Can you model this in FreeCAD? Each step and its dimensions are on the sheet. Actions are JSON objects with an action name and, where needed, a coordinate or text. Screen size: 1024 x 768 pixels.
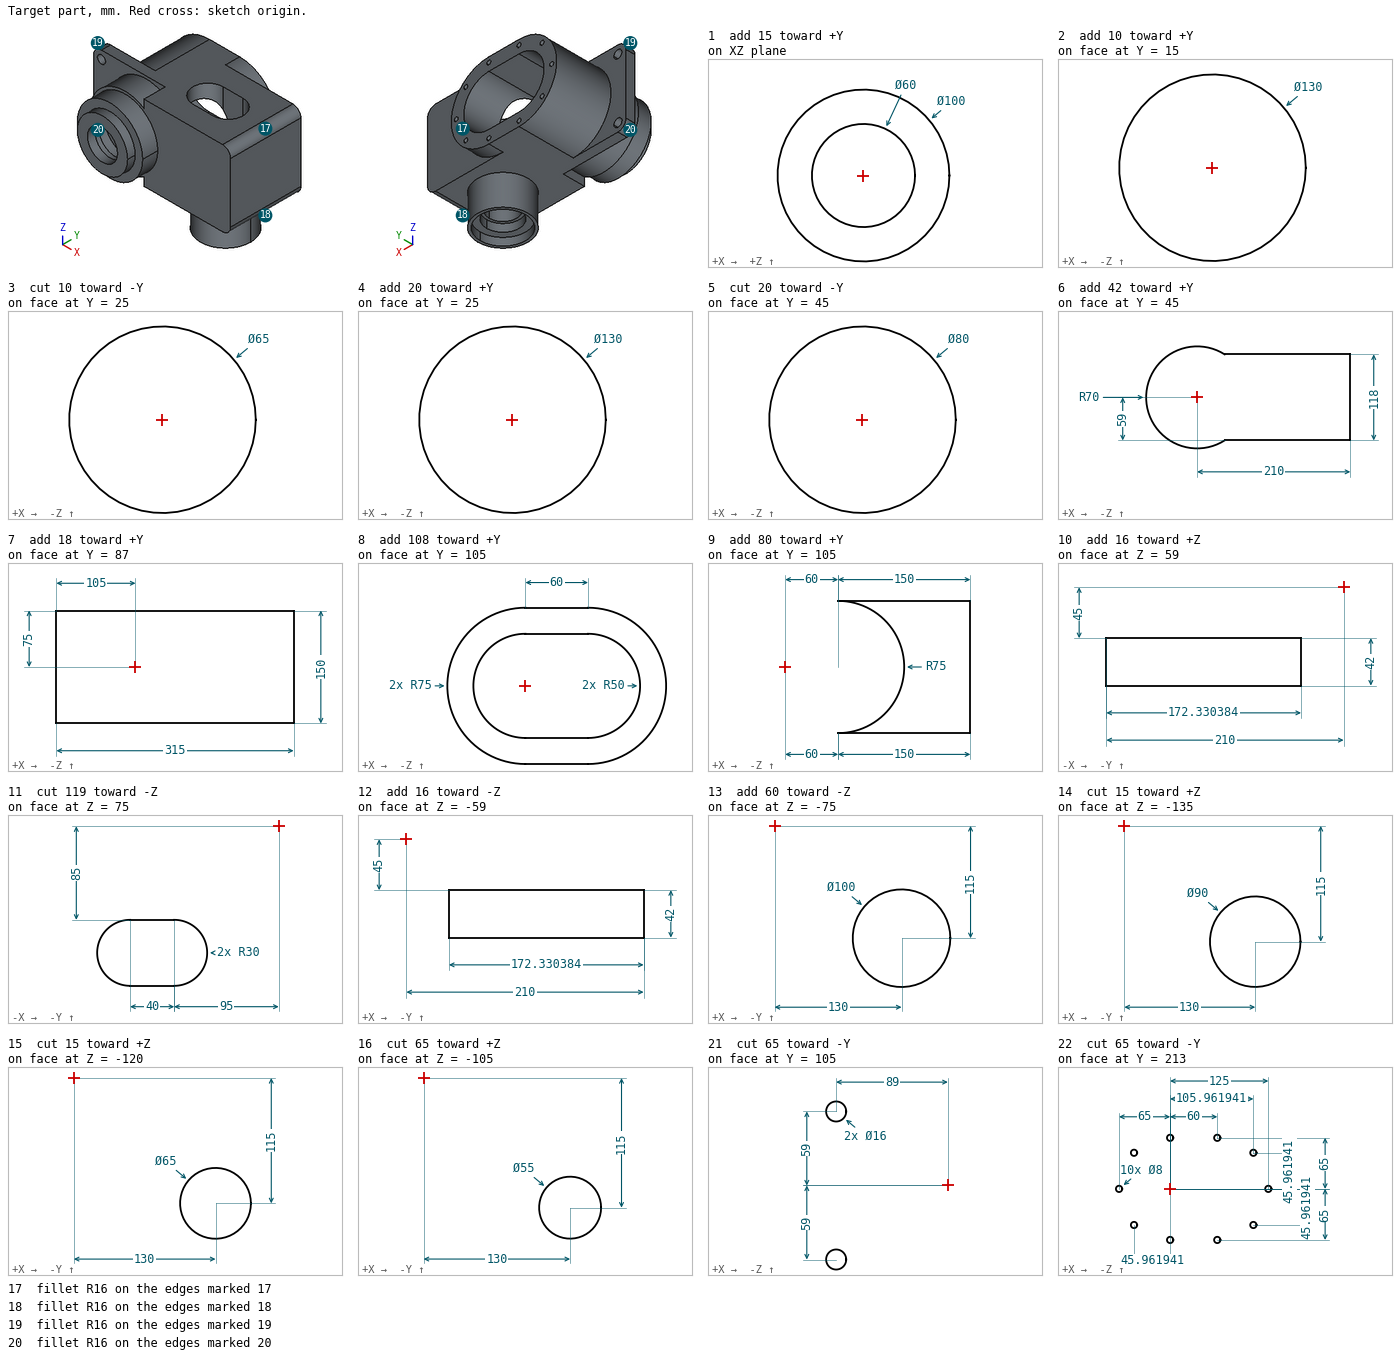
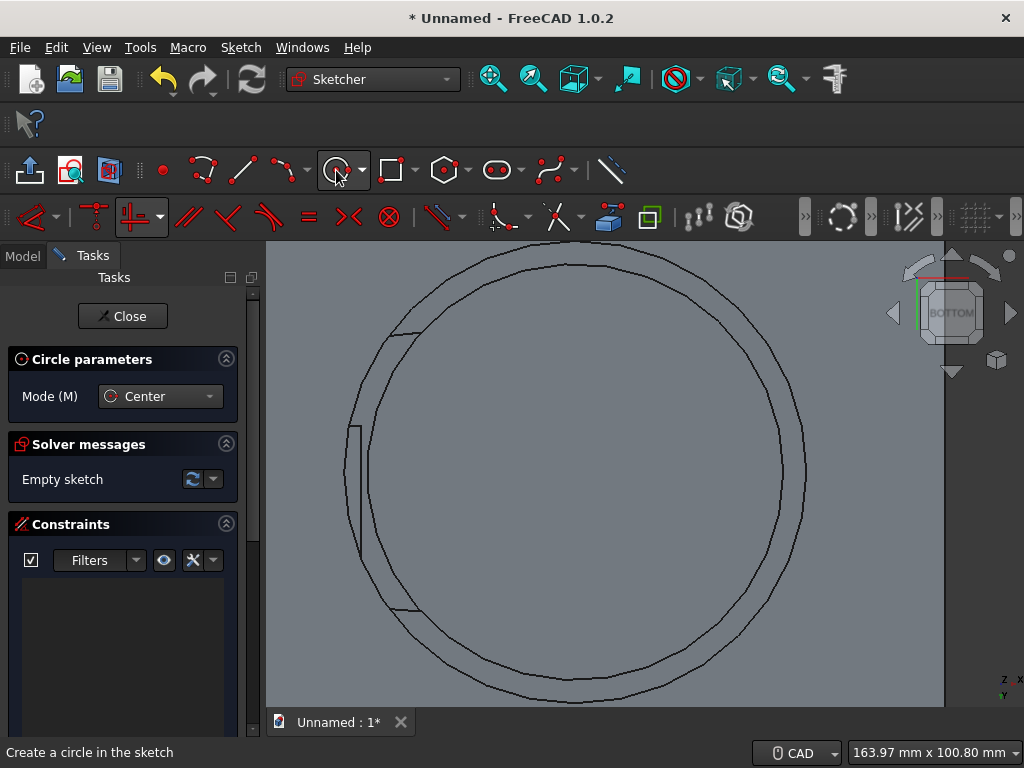
{"action": "left_click", "coordinate": [575, 472]}
{"action": "mouse_move", "coordinate": [682, 366]}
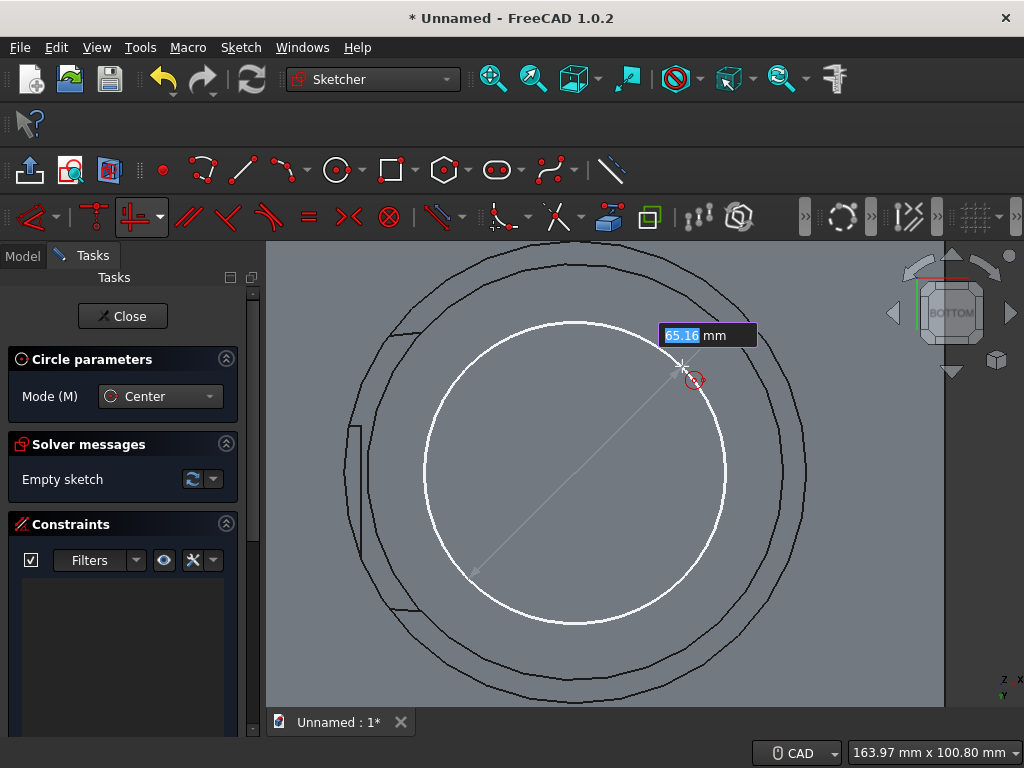
{"action": "type", "text": "65"}
{"action": "key", "text": "Return"}
{"action": "key", "text": "Escape"}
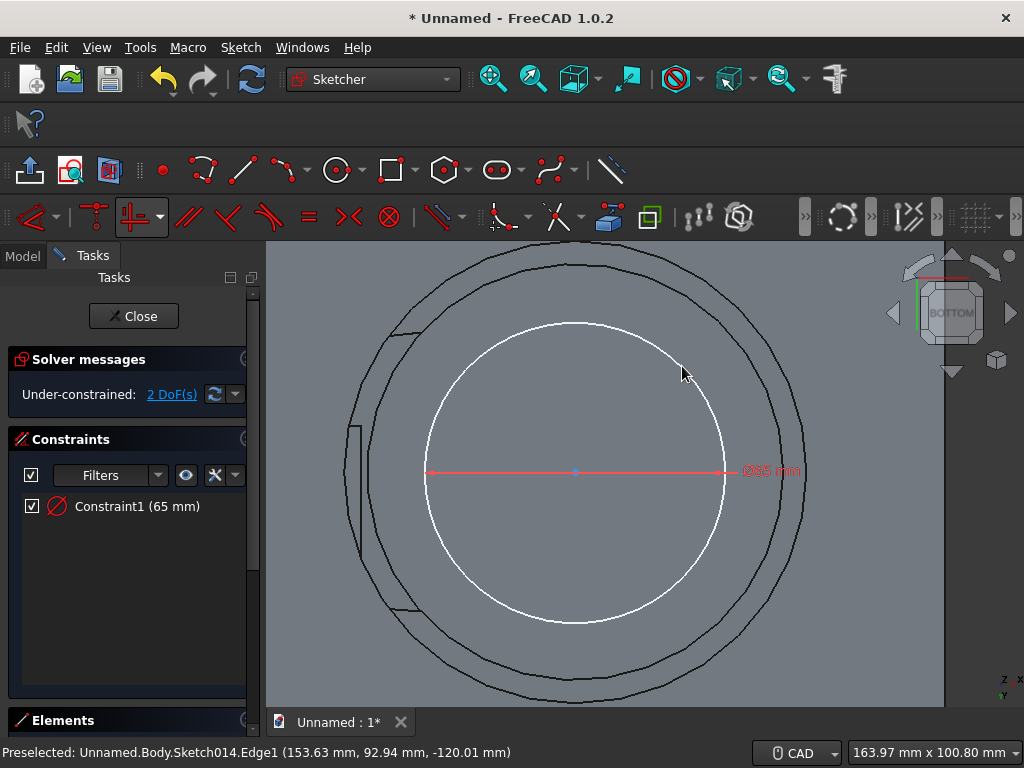
{"action": "left_click", "coordinate": [32, 218]}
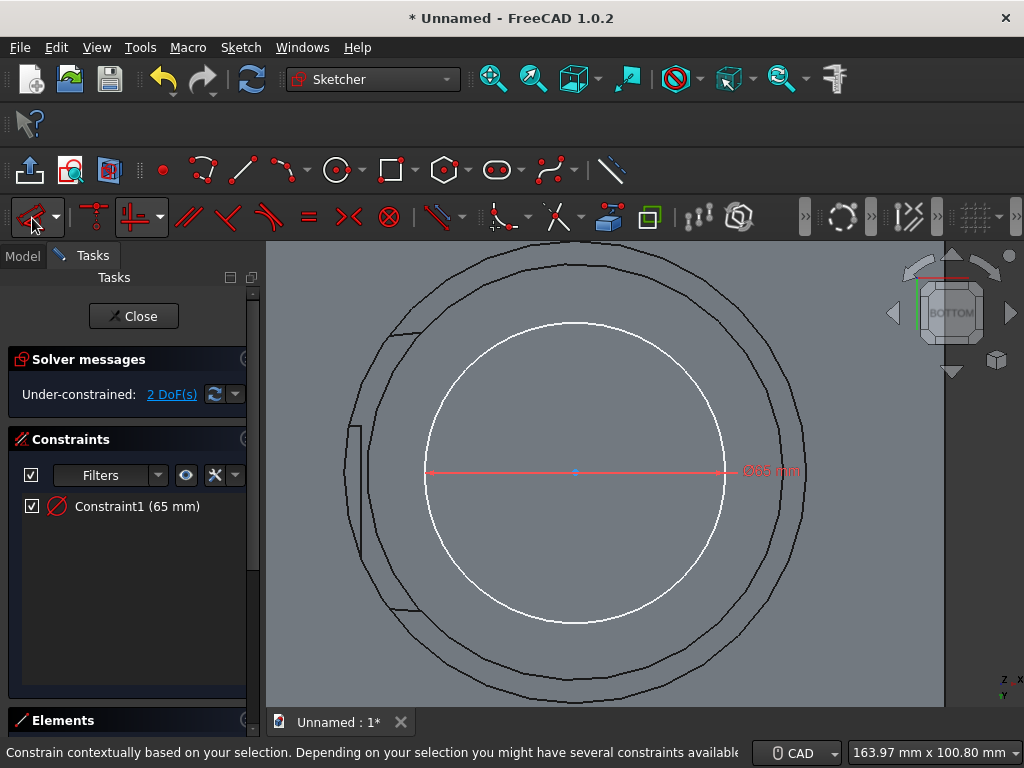
{"action": "left_click", "coordinate": [575, 473]}
{"action": "left_click", "coordinate": [370, 507]}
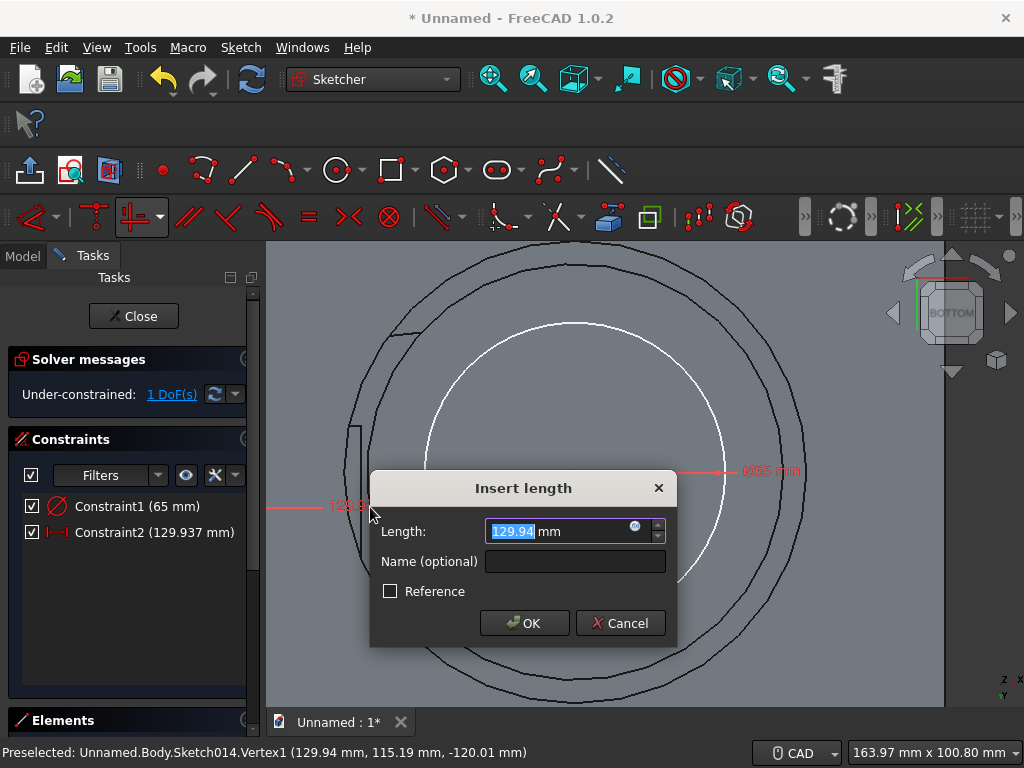
{"action": "type", "text": "130"}
{"action": "key", "text": "Return"}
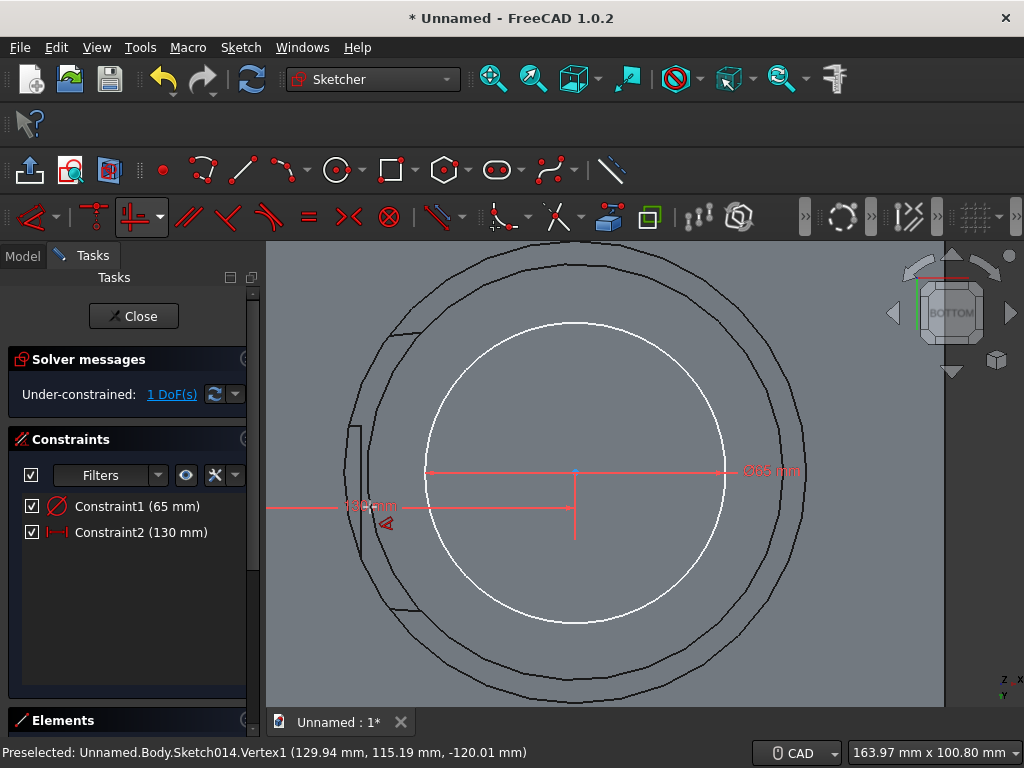
{"action": "left_click", "coordinate": [575, 473]}
{"action": "left_click", "coordinate": [609, 371]}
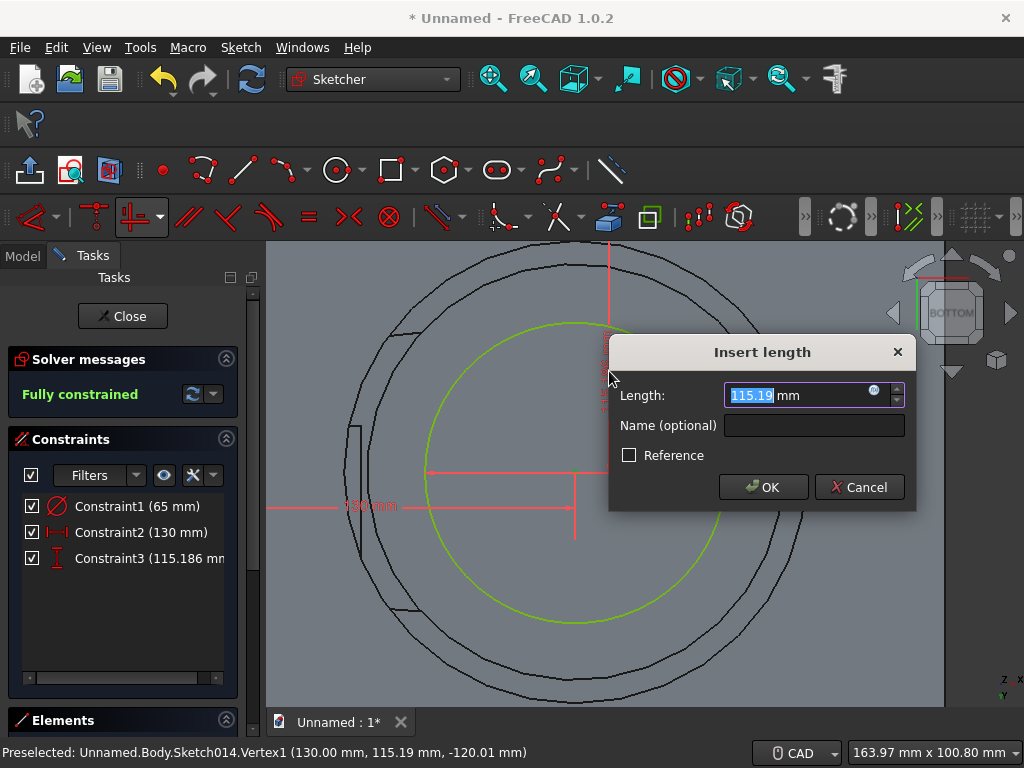
{"action": "type", "text": "115"}
{"action": "key", "text": "Return"}
{"action": "key", "text": "Escape"}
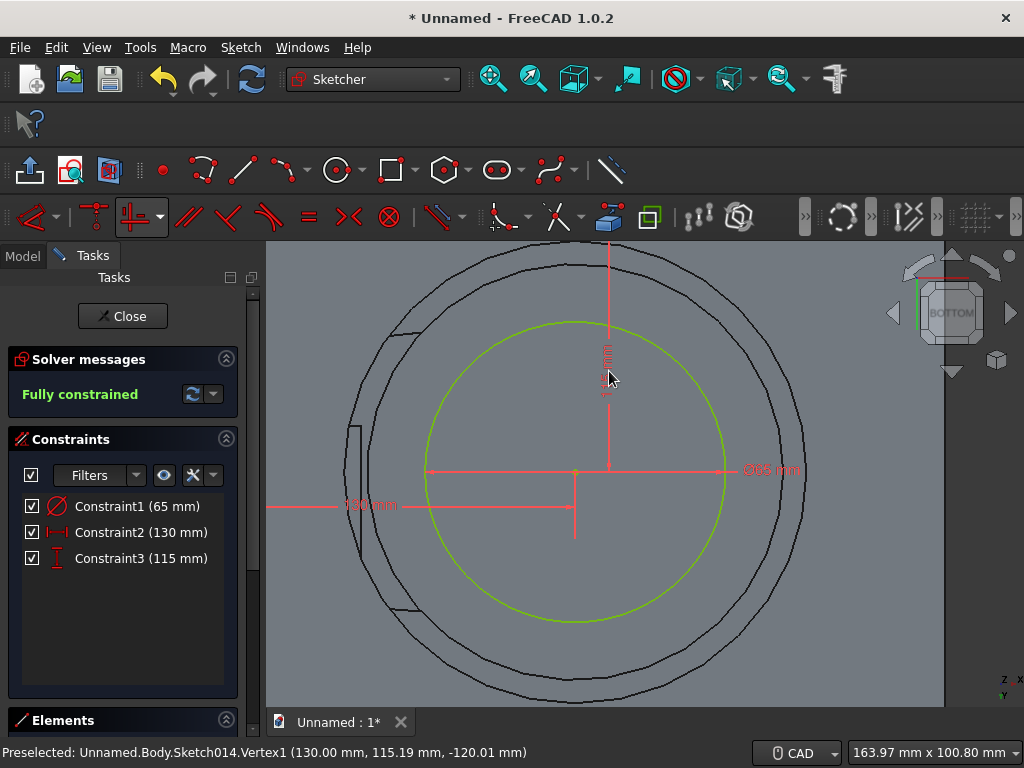
{"action": "left_click", "coordinate": [123, 316]}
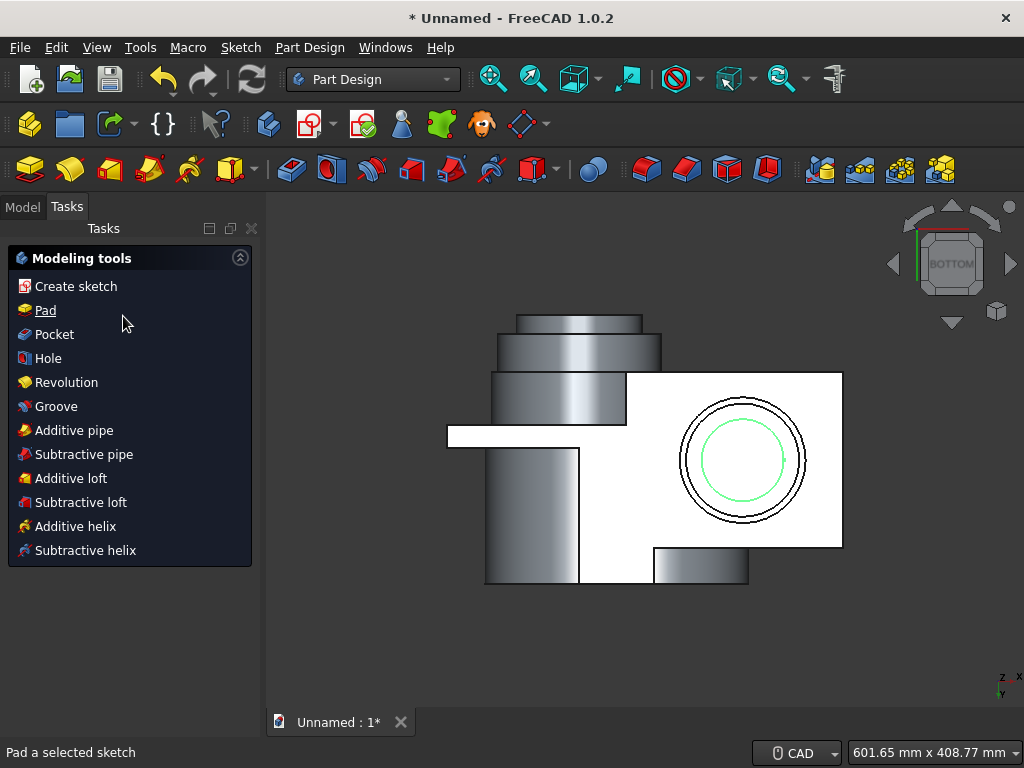
{"action": "left_click", "coordinate": [292, 170]}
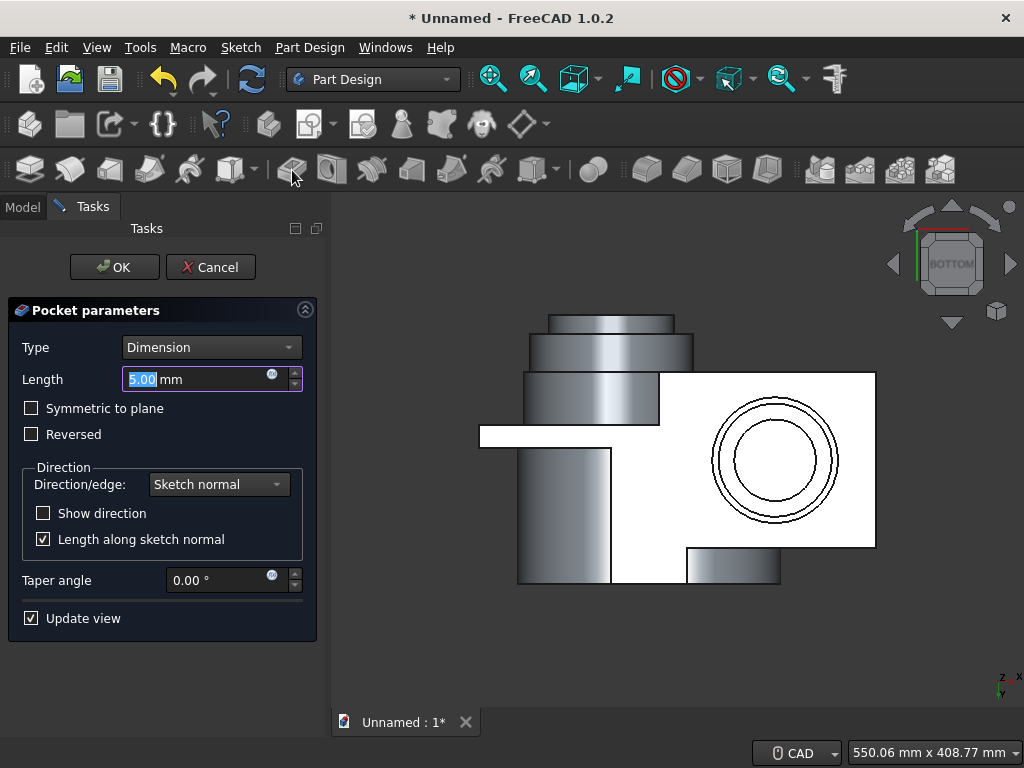
{"action": "type", "text": "15"}
{"action": "key", "text": "Tab"}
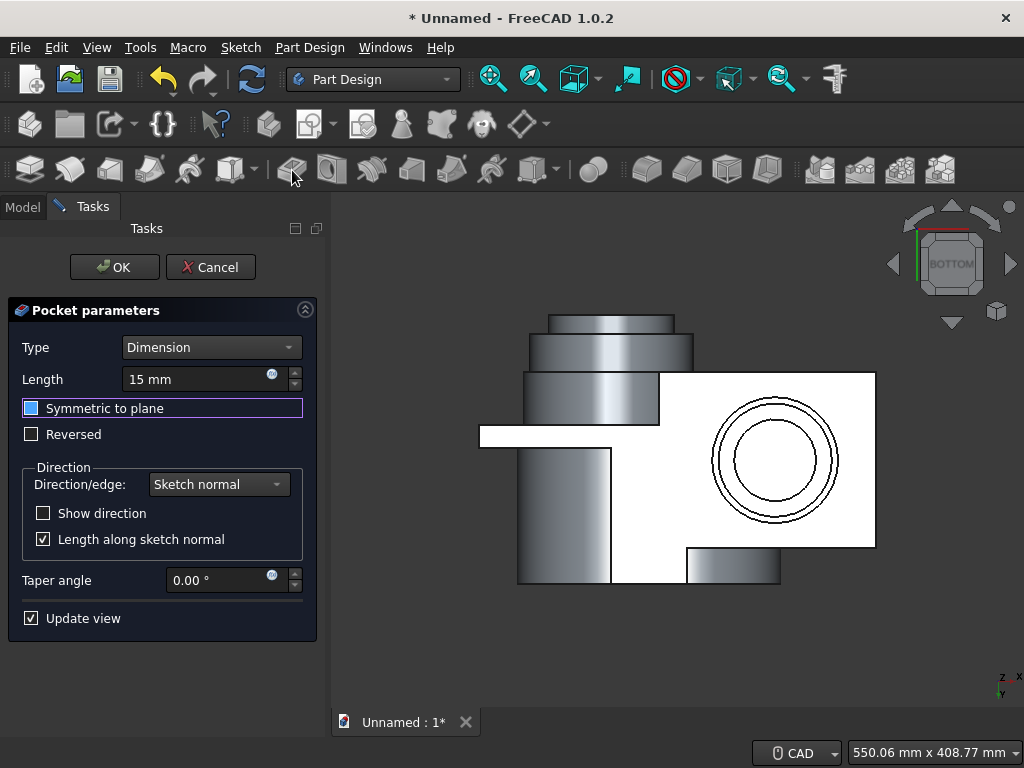
{"action": "left_click", "coordinate": [115, 267]}